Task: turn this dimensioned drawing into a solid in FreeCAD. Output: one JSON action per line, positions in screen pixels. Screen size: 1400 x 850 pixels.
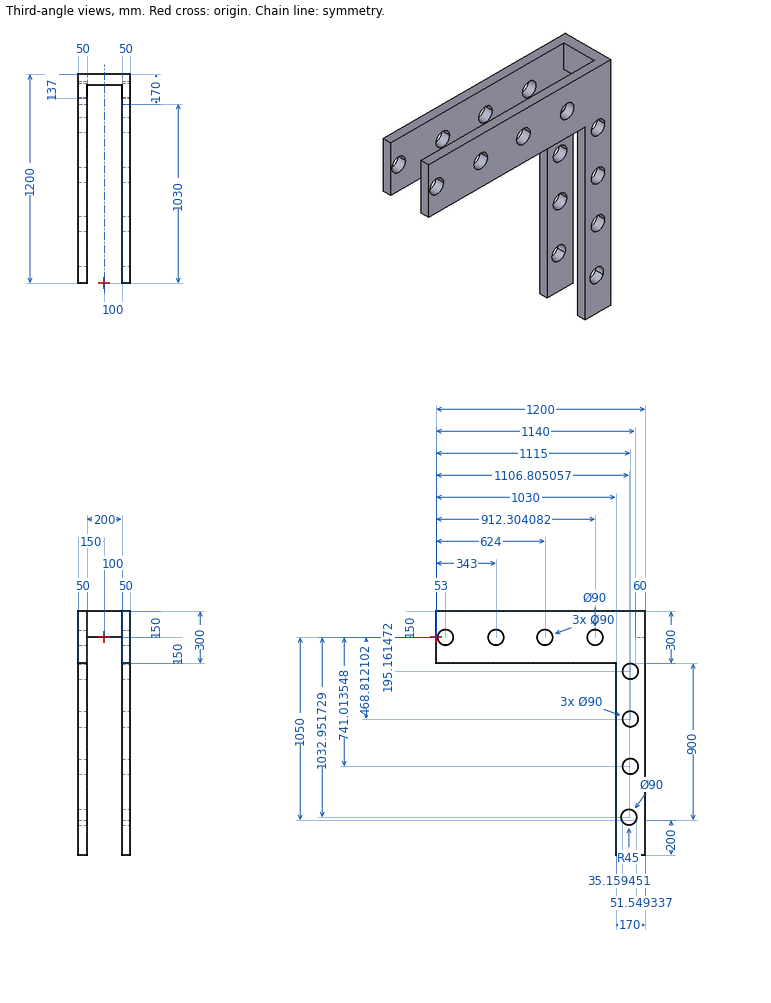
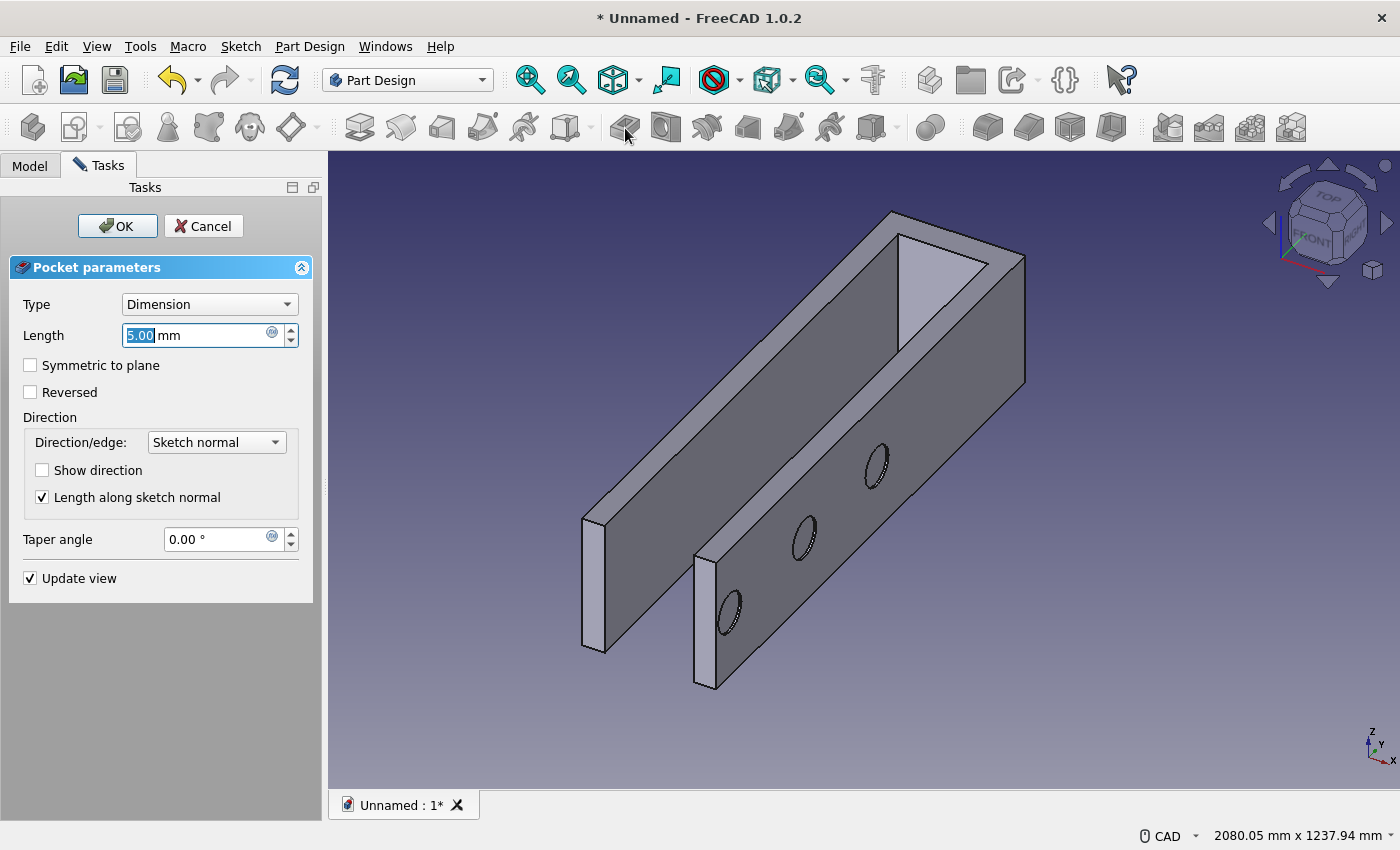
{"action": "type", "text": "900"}
{"action": "key", "text": "Tab"}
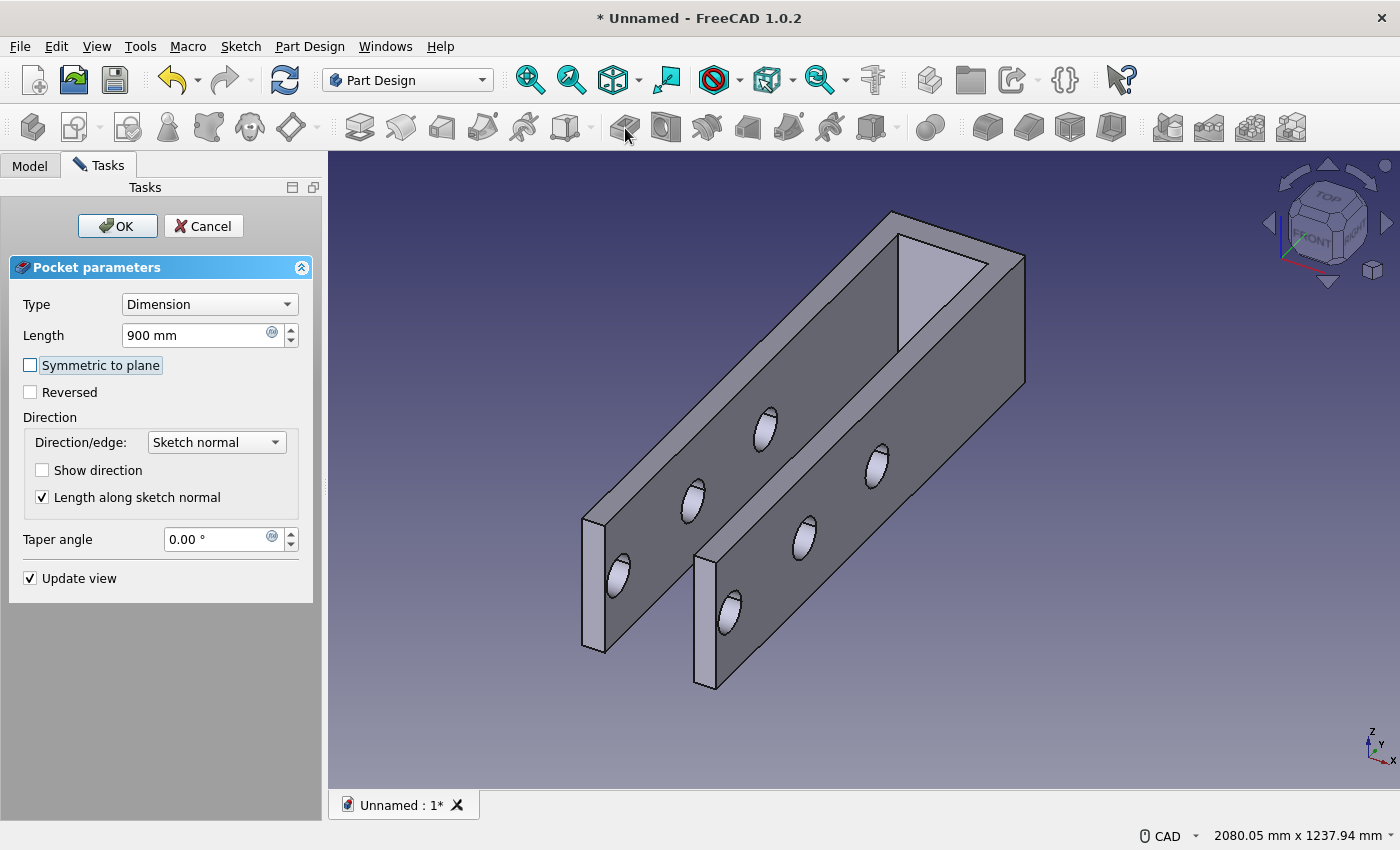
{"action": "left_click", "coordinate": [118, 226]}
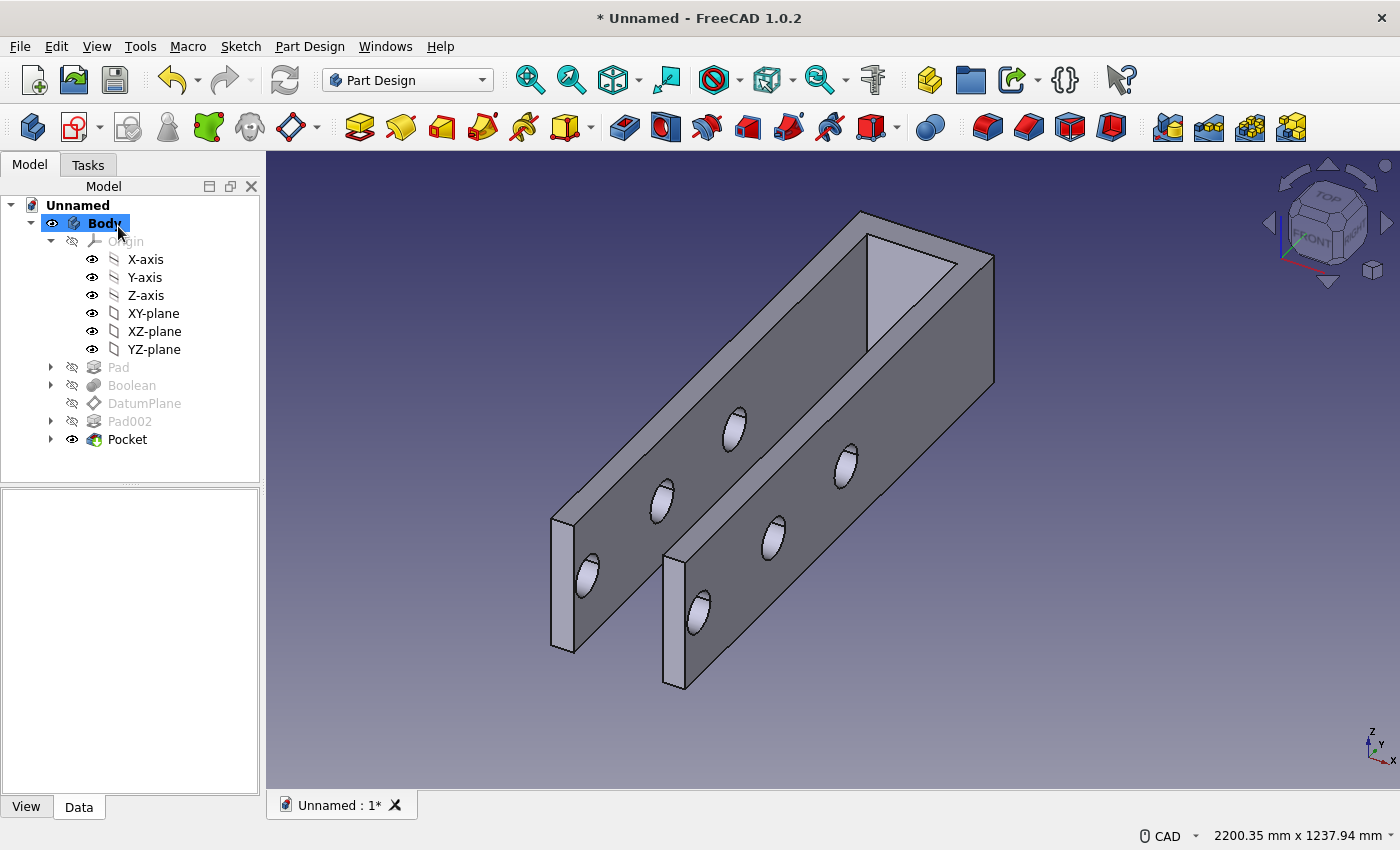
{"action": "key", "text": "5"}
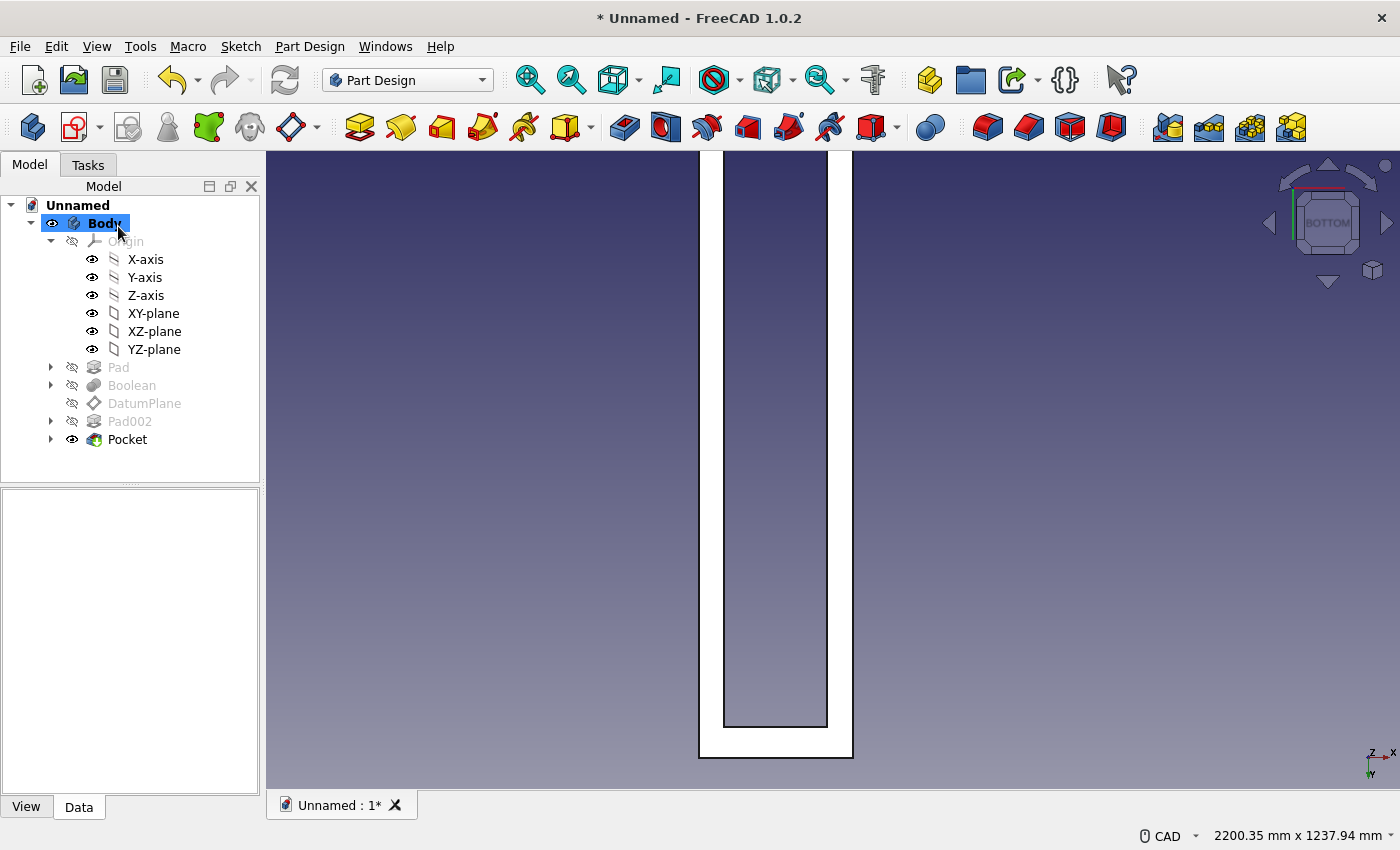
{"action": "left_click", "coordinate": [531, 80]}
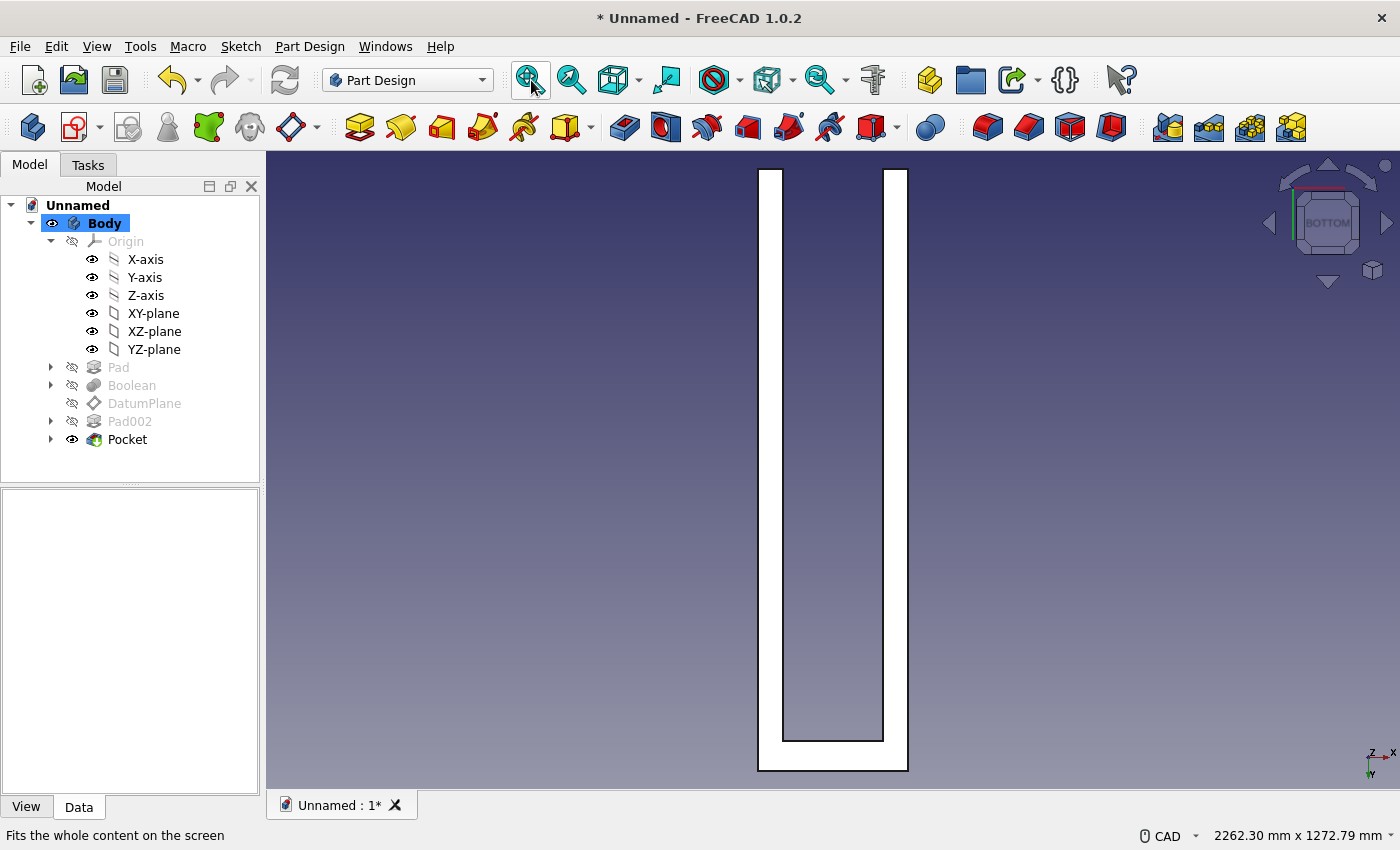
{"action": "left_click", "coordinate": [769, 727]}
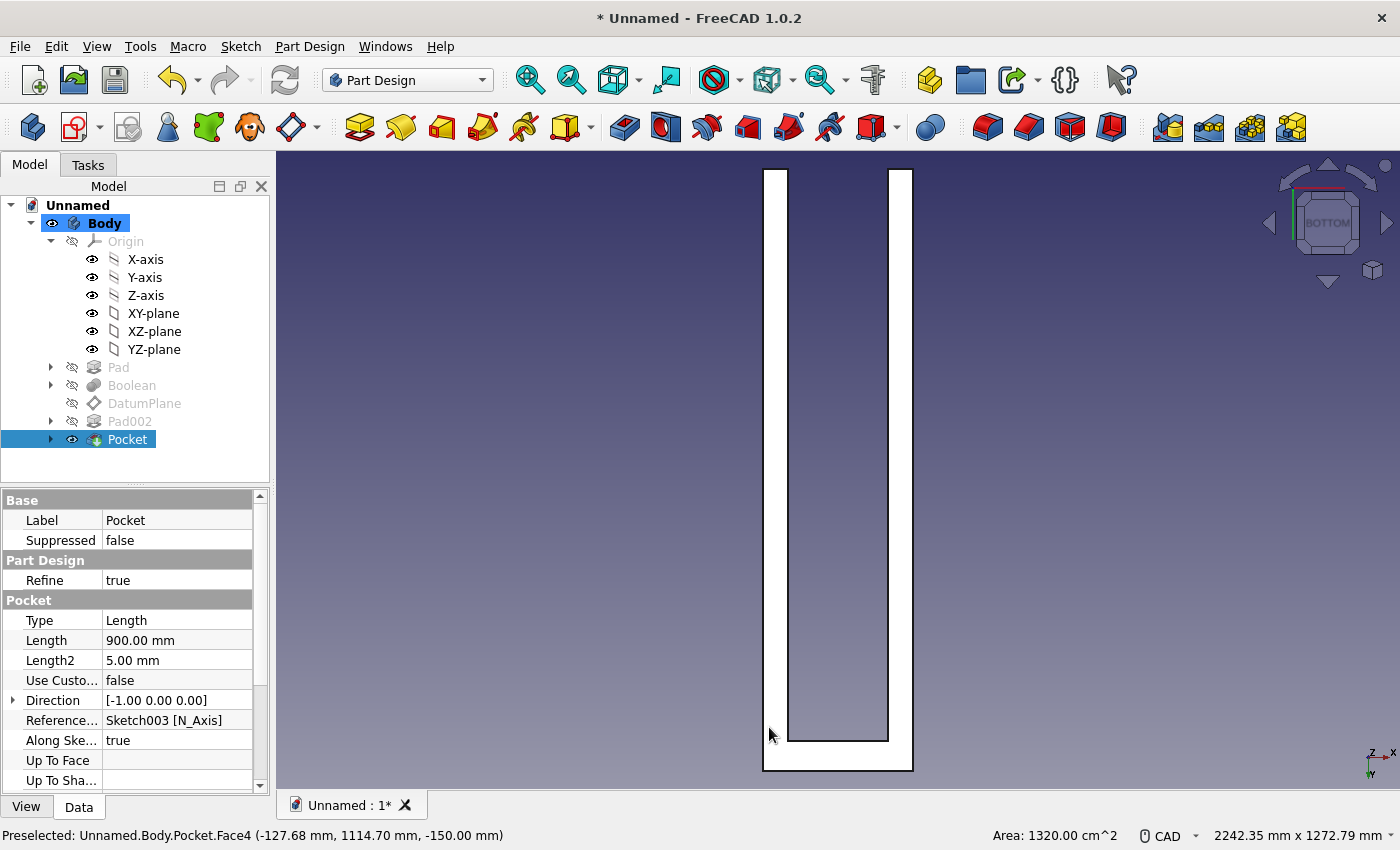
{"action": "left_click", "coordinate": [74, 128]}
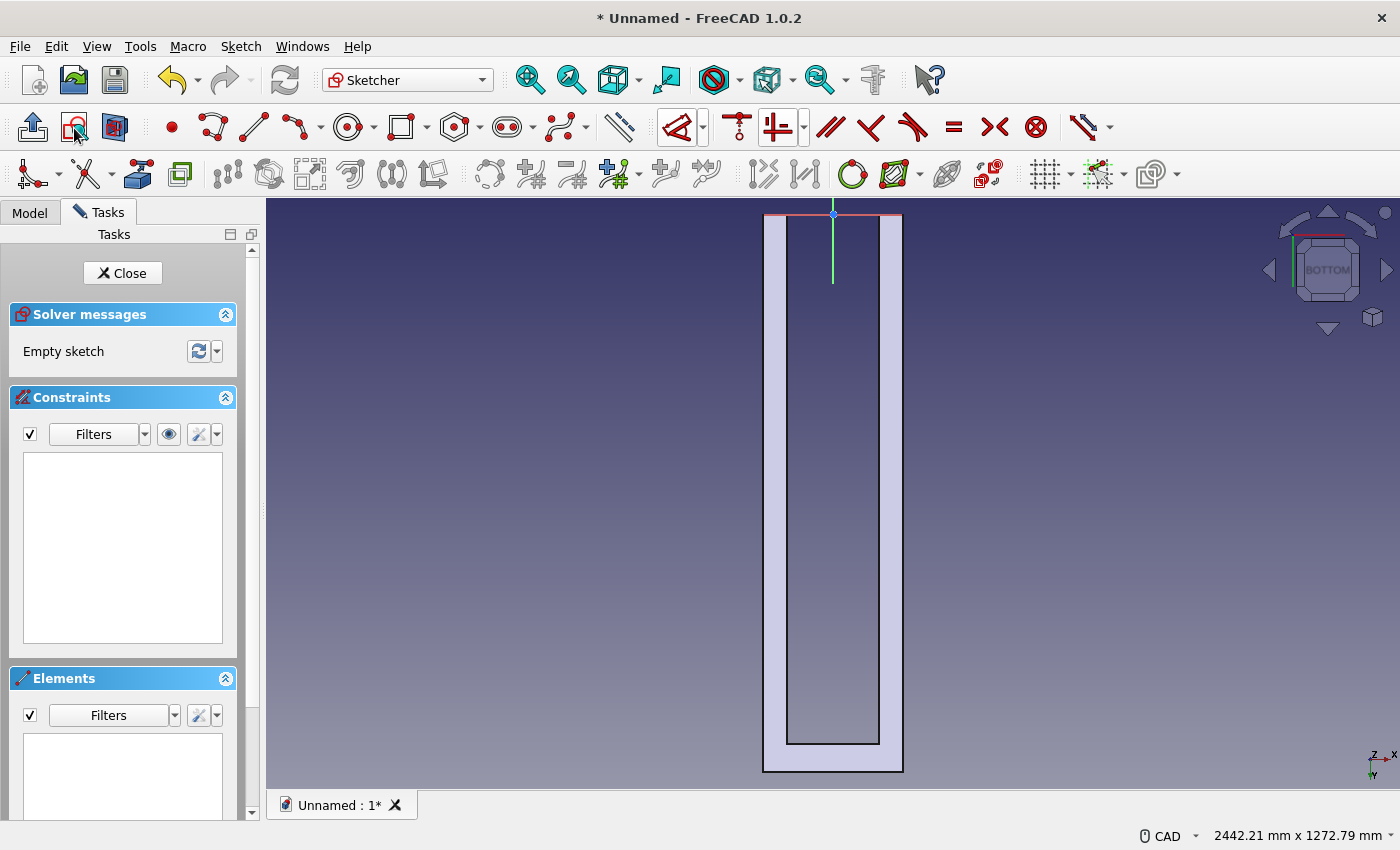
{"action": "scroll", "coordinate": [764, 494], "scroll_direction": "down", "scroll_amount": 5}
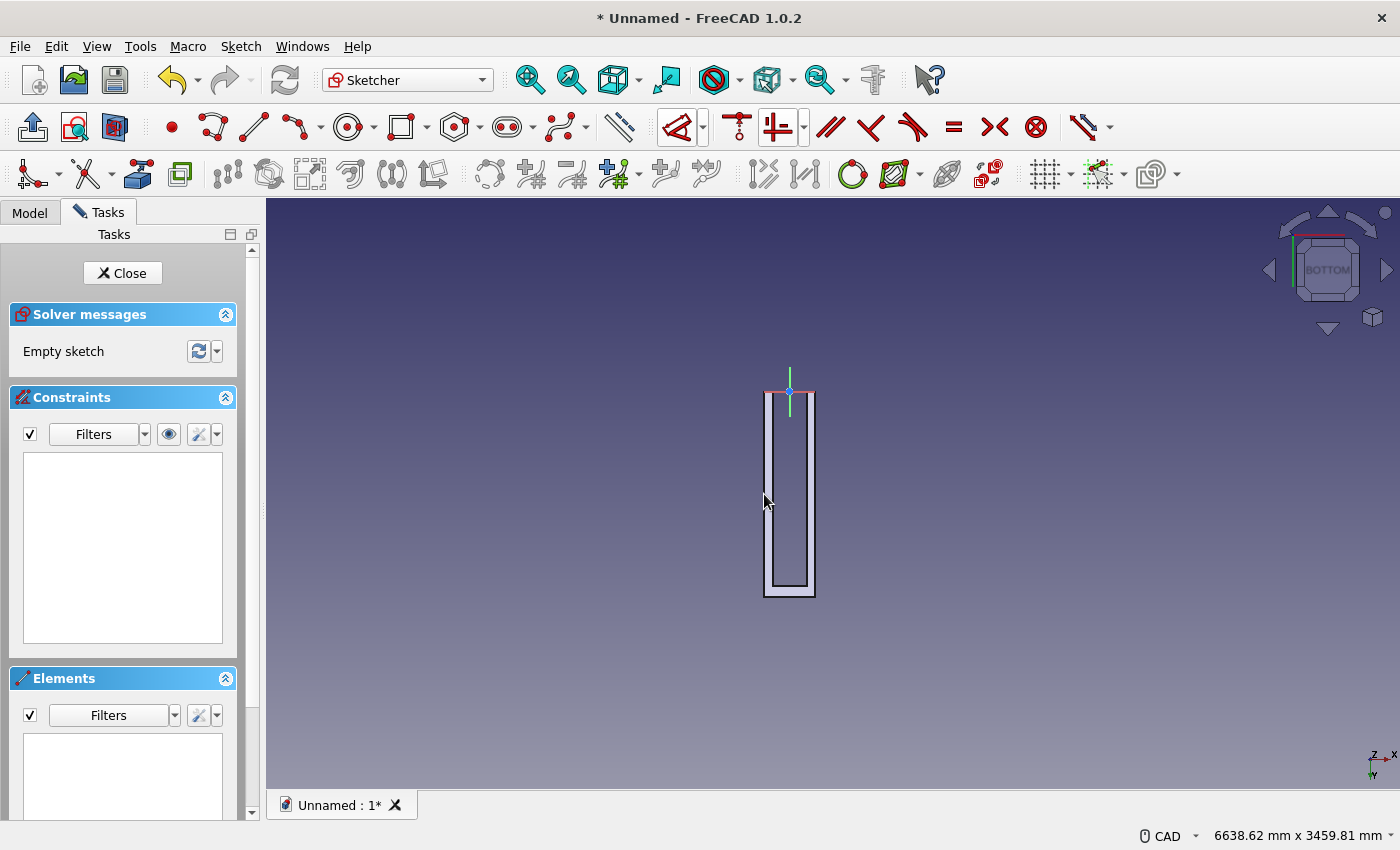
{"action": "scroll", "coordinate": [792, 589], "scroll_direction": "up", "scroll_amount": 13}